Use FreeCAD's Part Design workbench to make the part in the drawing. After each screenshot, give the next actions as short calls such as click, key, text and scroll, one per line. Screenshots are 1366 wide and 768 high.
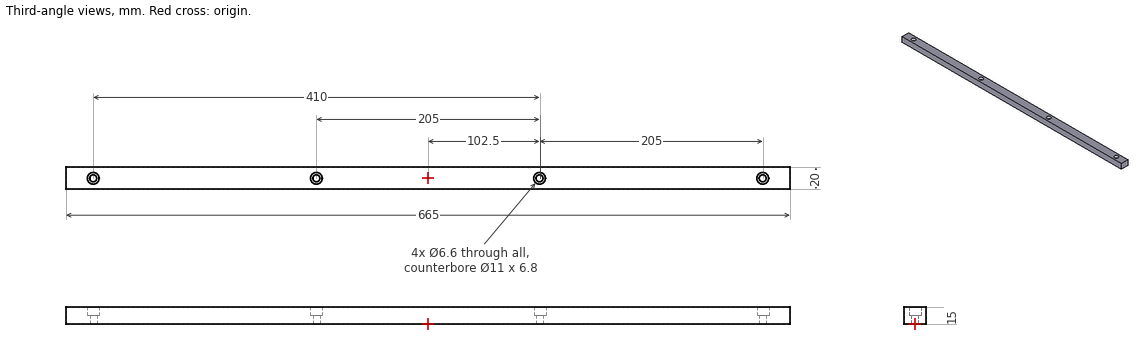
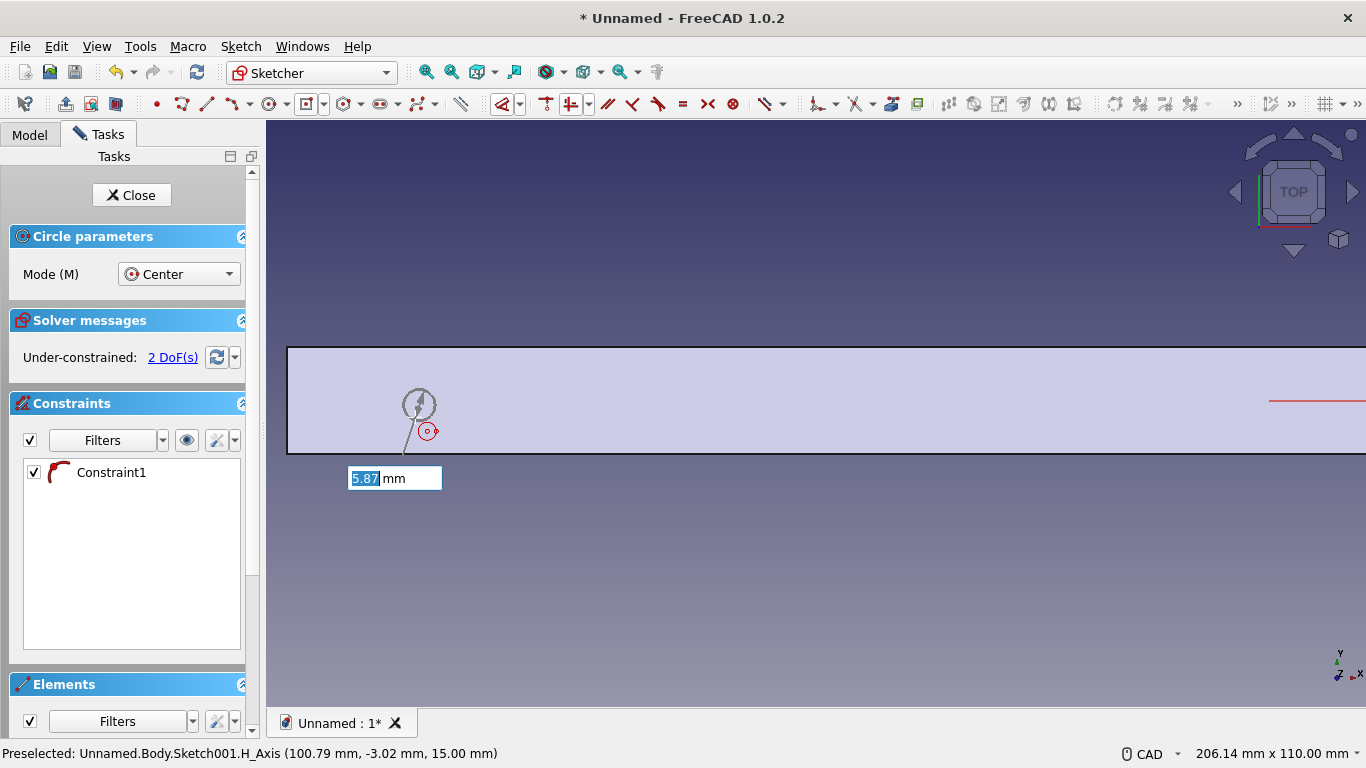
click(415, 417)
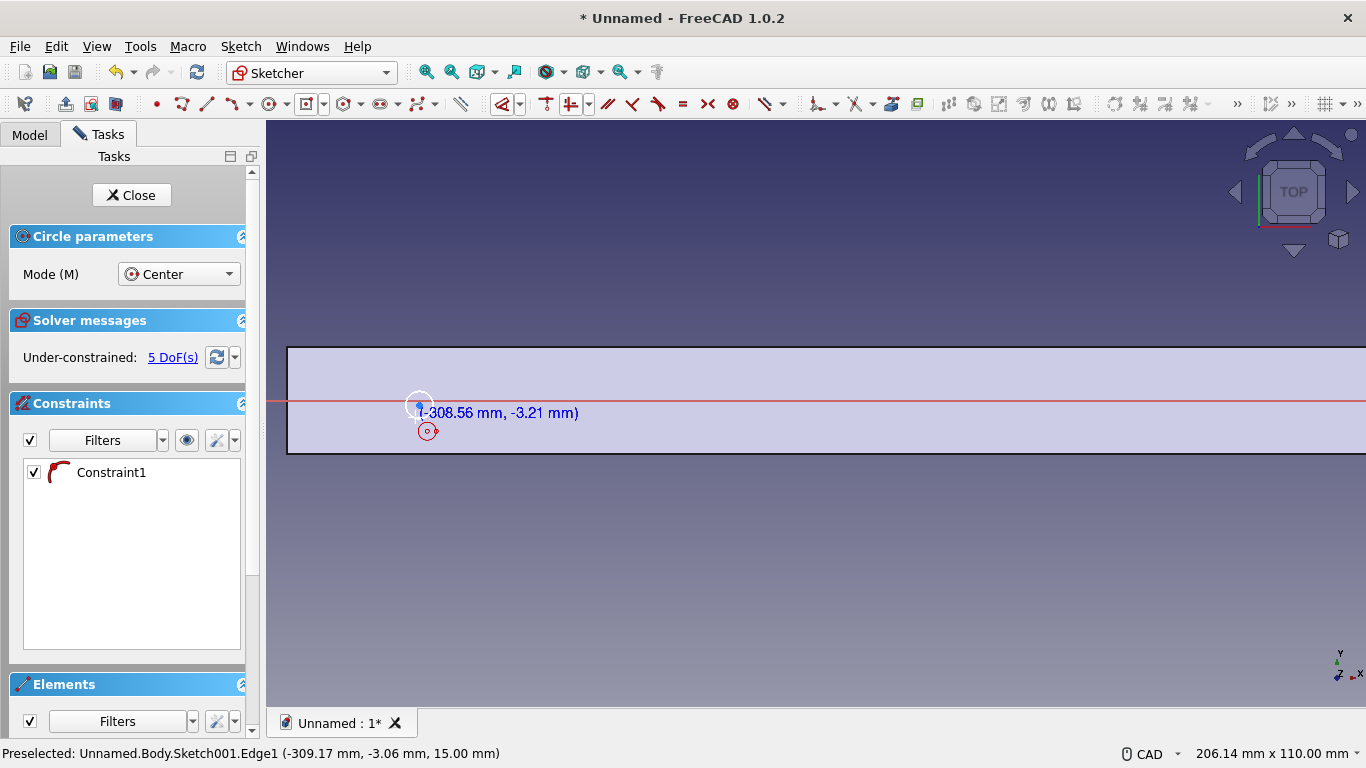
scroll(415, 417, down, 8)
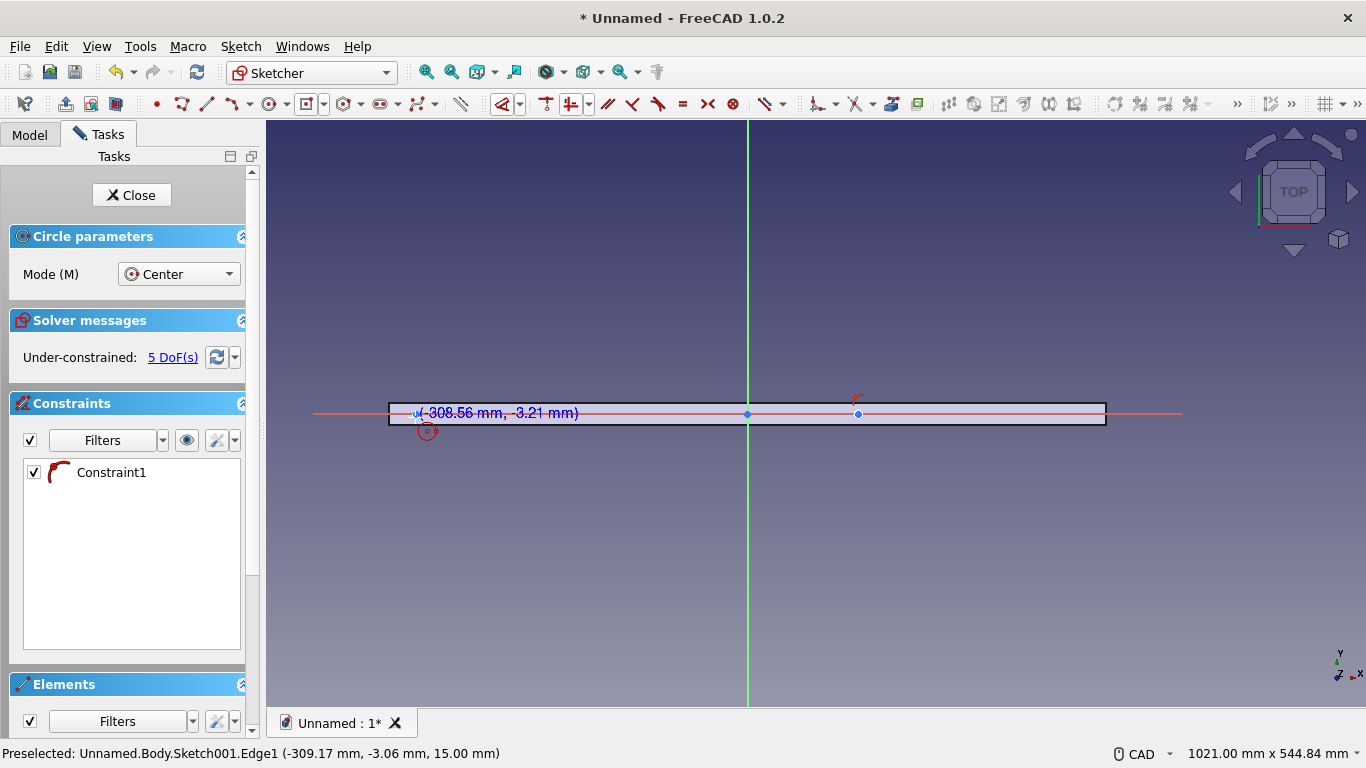
scroll(1079, 414, up, 10)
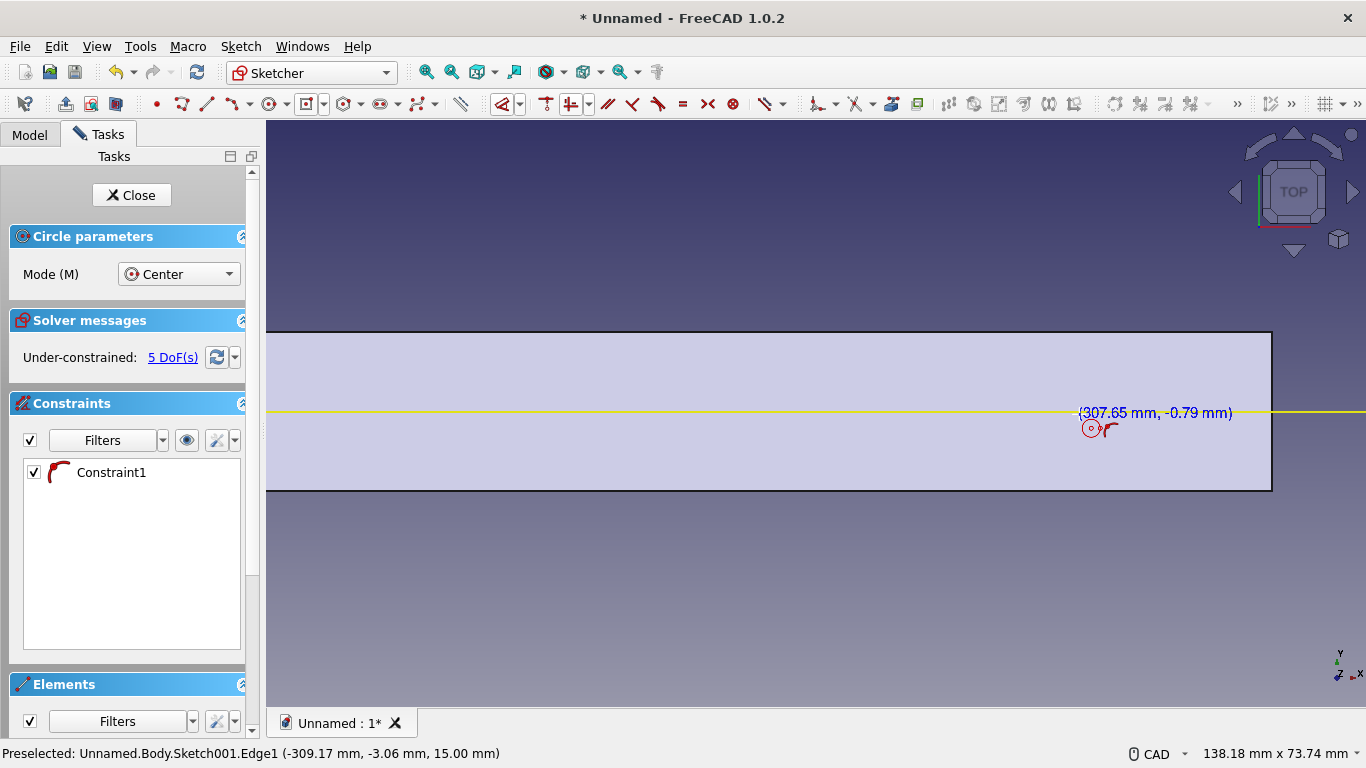
scroll(1080, 414, down, 10)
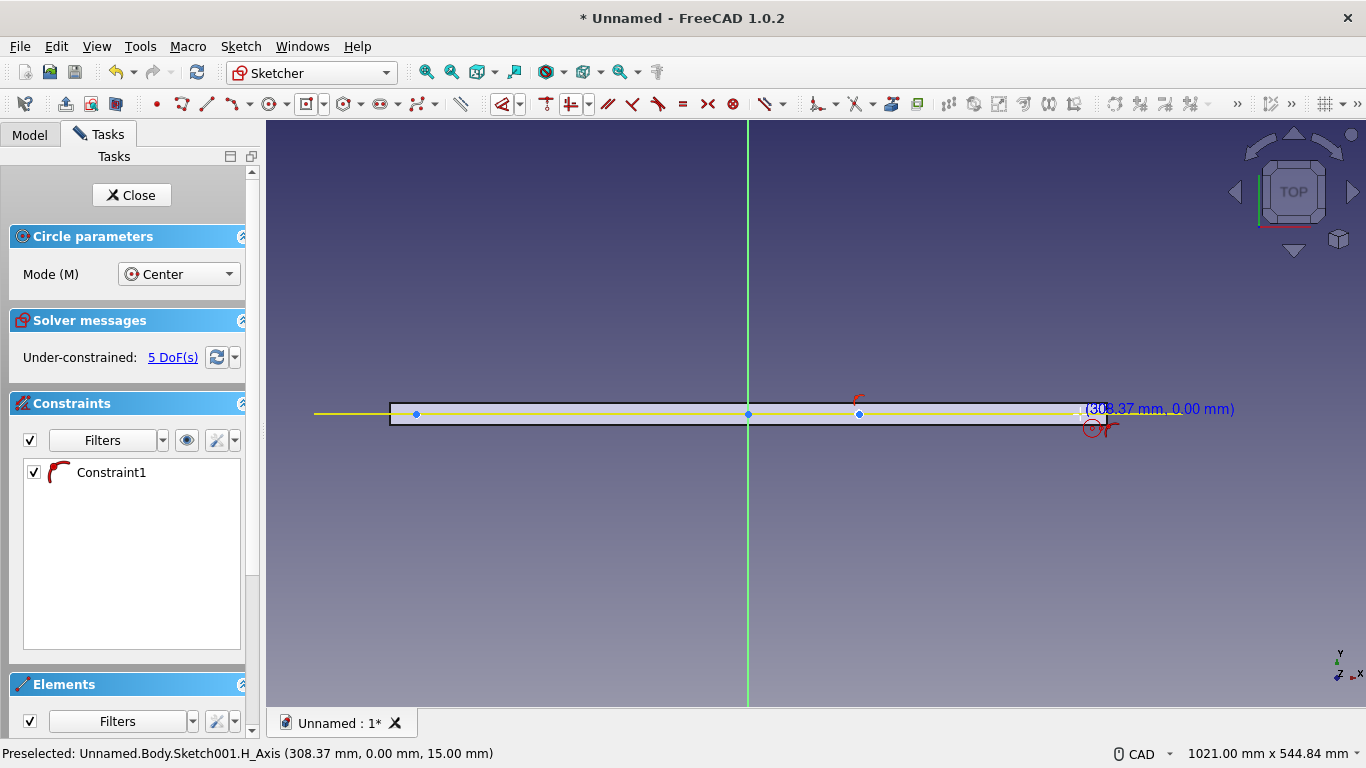
click(1080, 414)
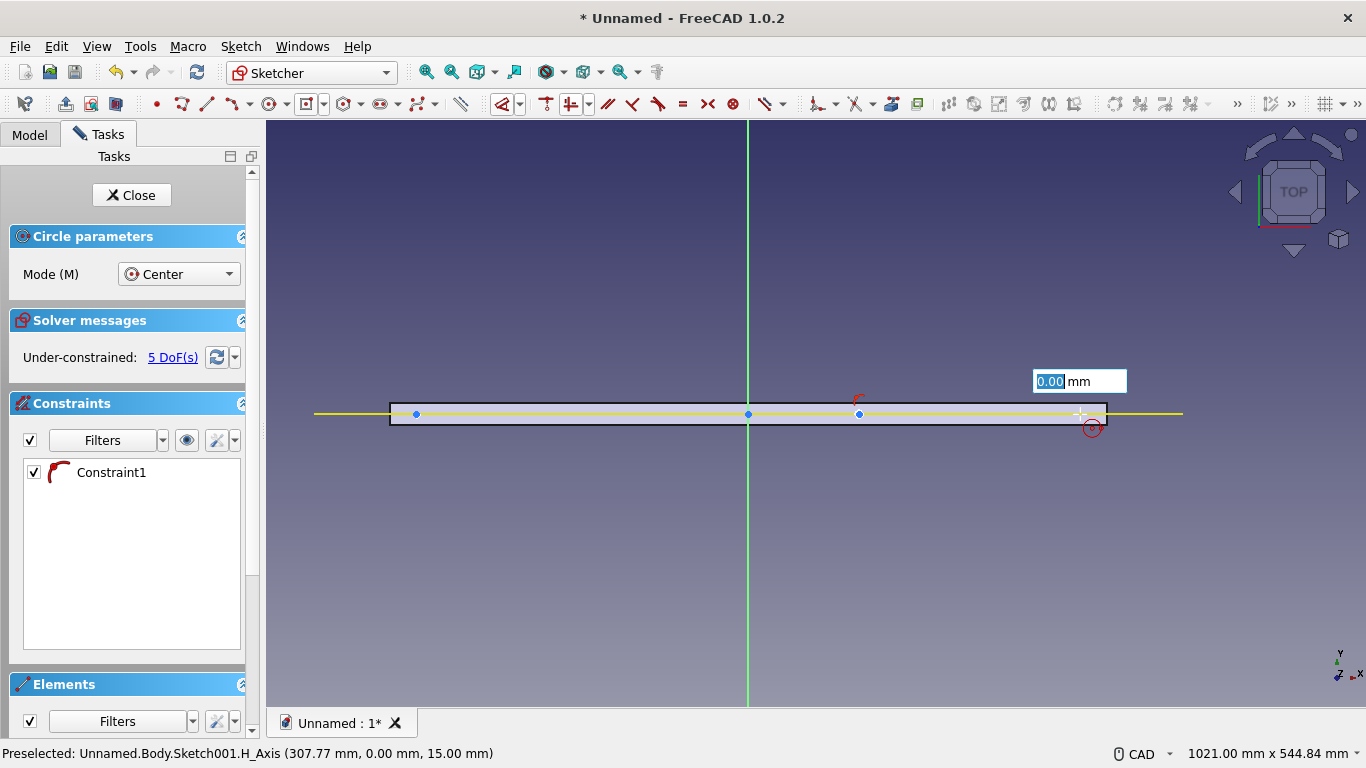
scroll(1078, 417, up, 8)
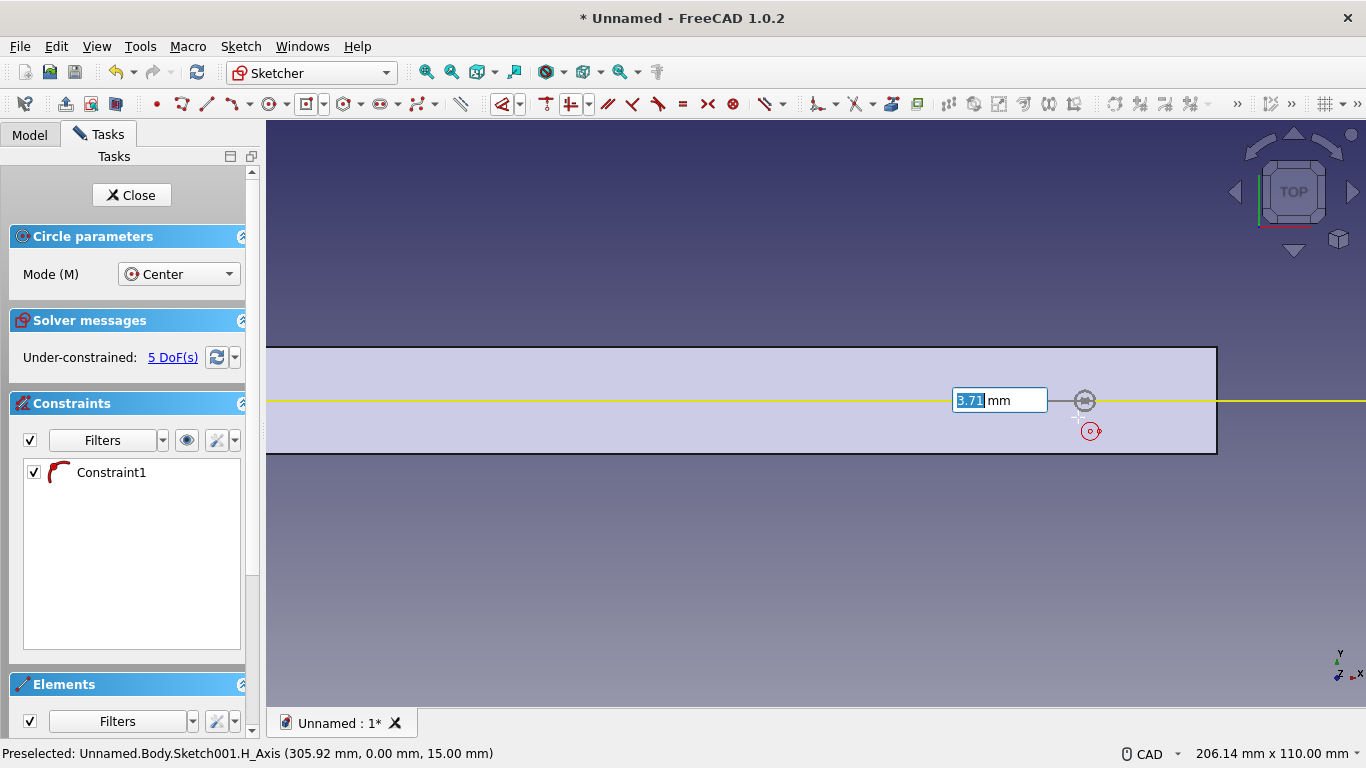
click(1078, 417)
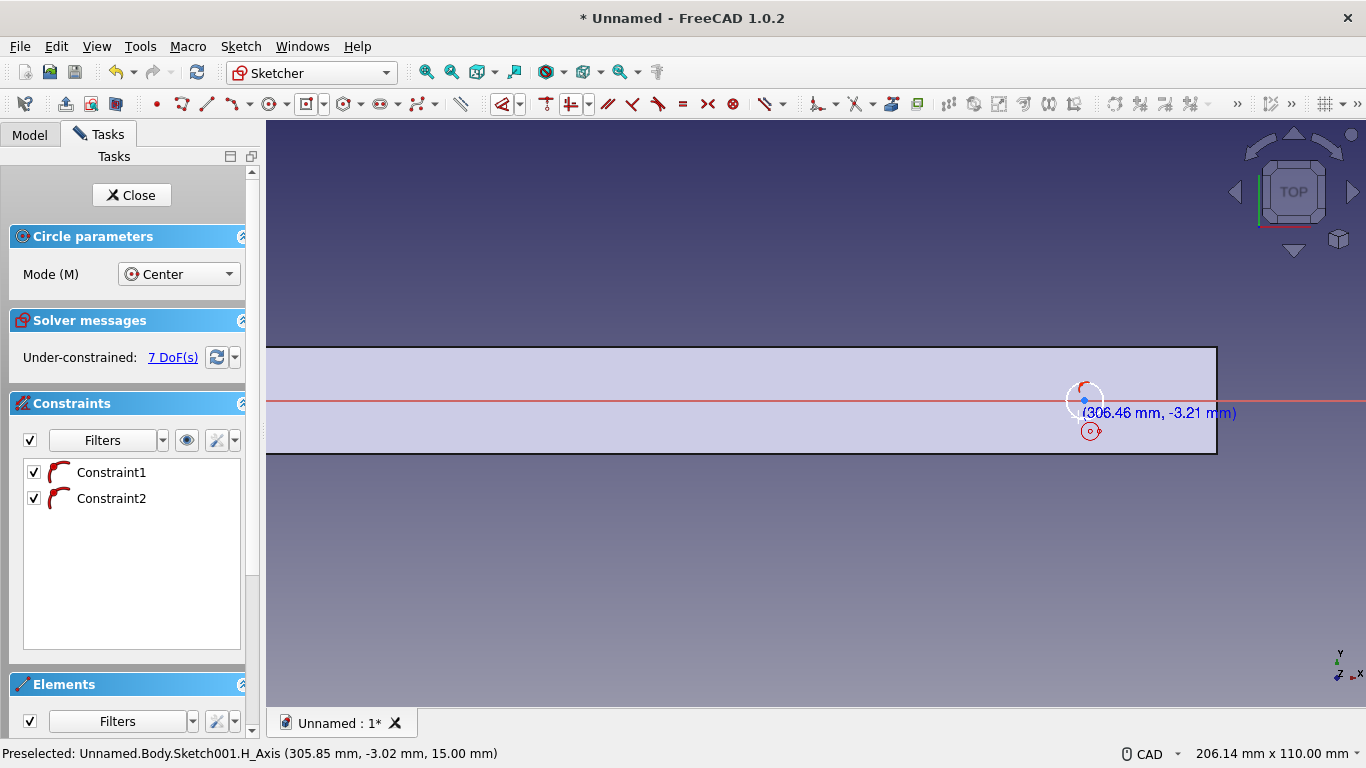
scroll(1078, 417, down, 8)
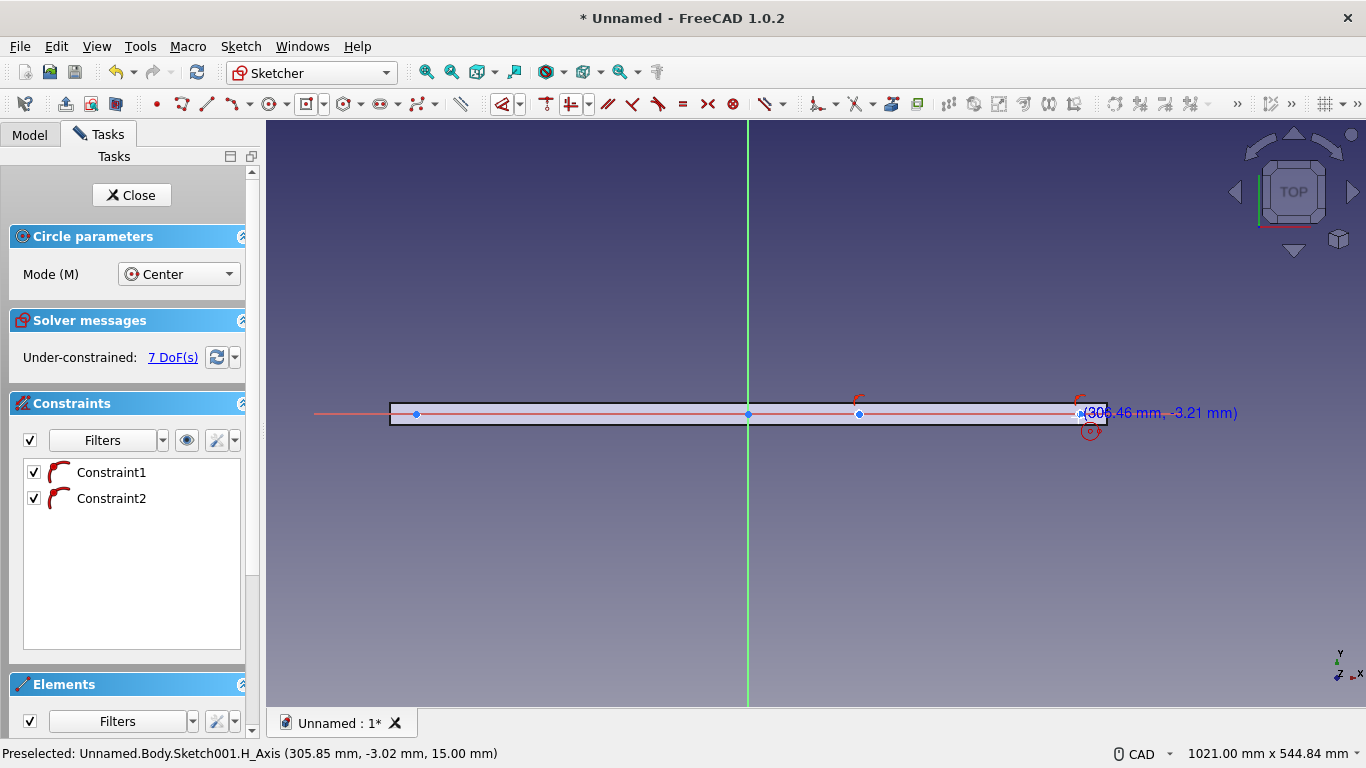
scroll(638, 414, up, 10)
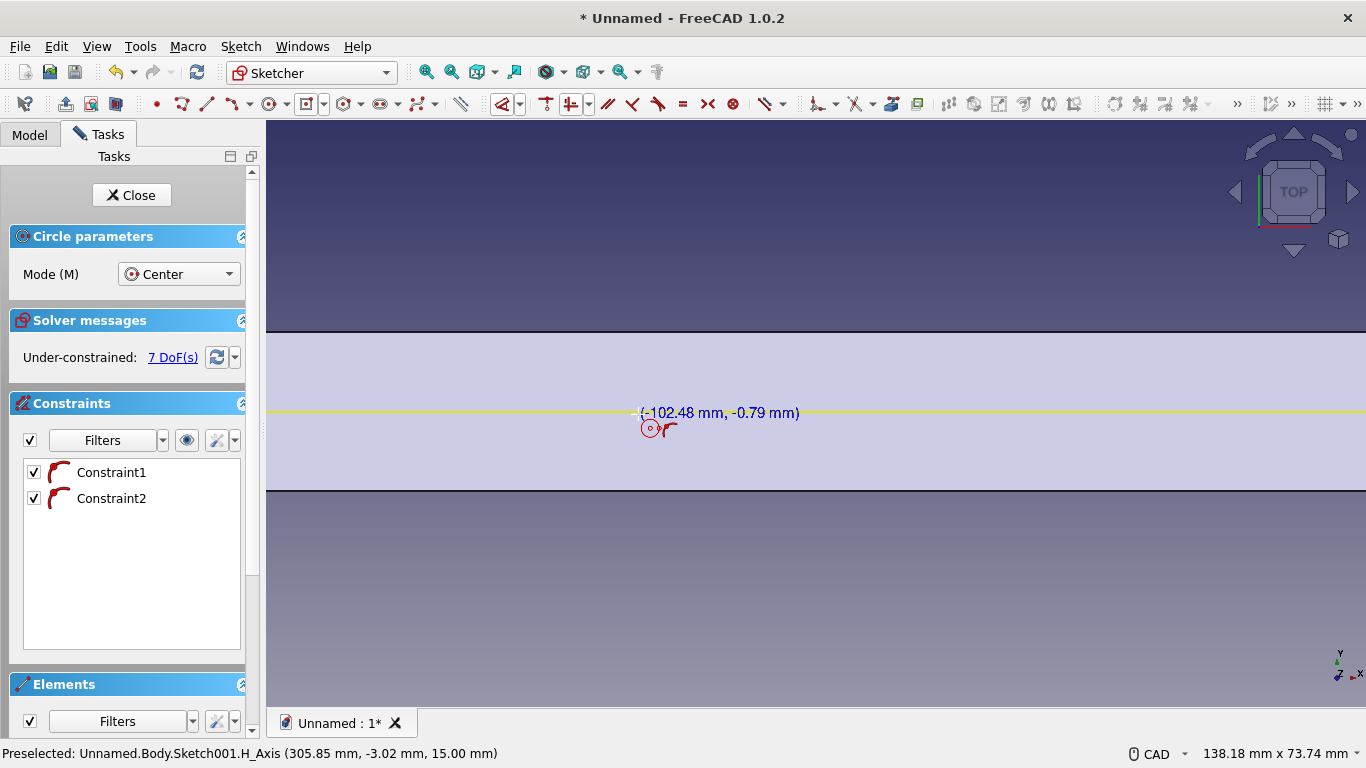
scroll(637, 414, down, 10)